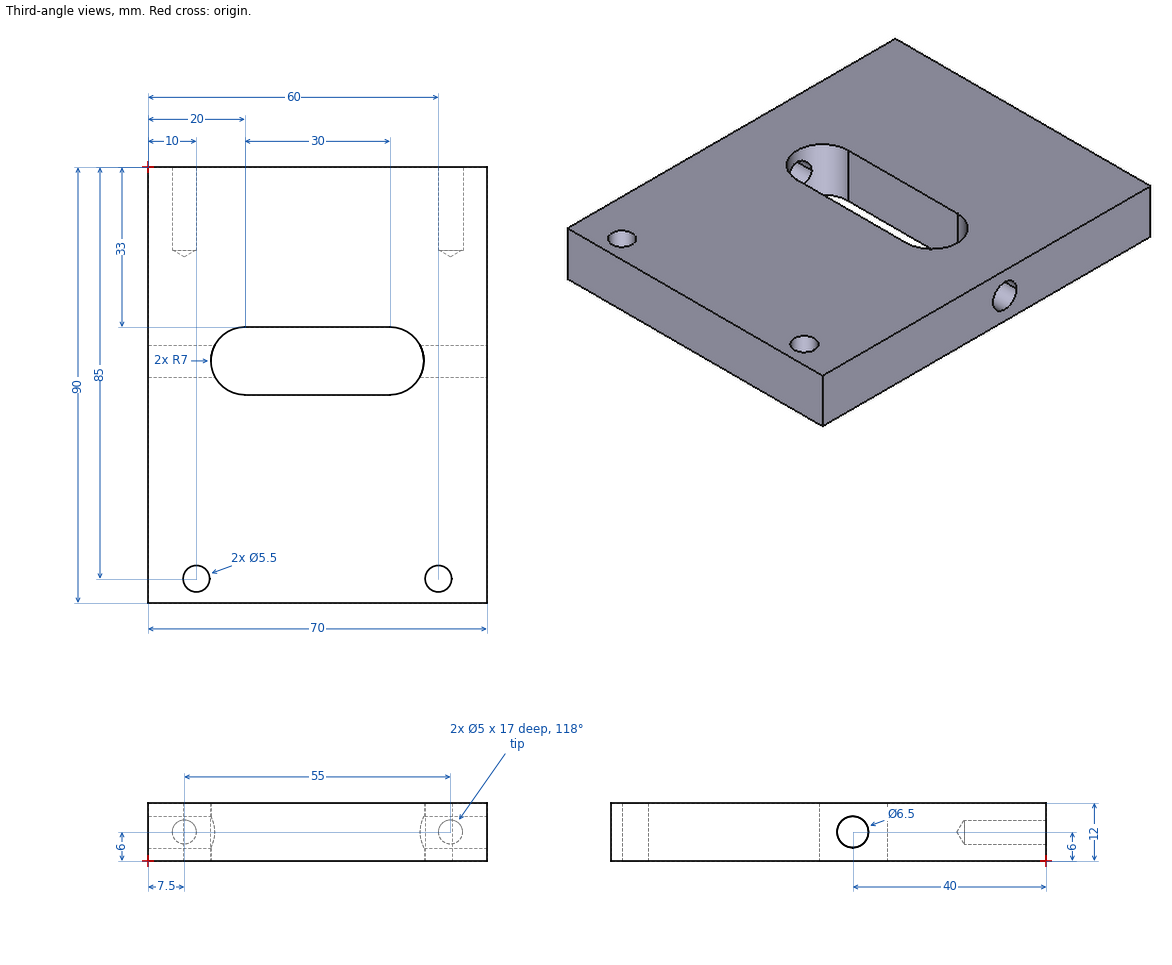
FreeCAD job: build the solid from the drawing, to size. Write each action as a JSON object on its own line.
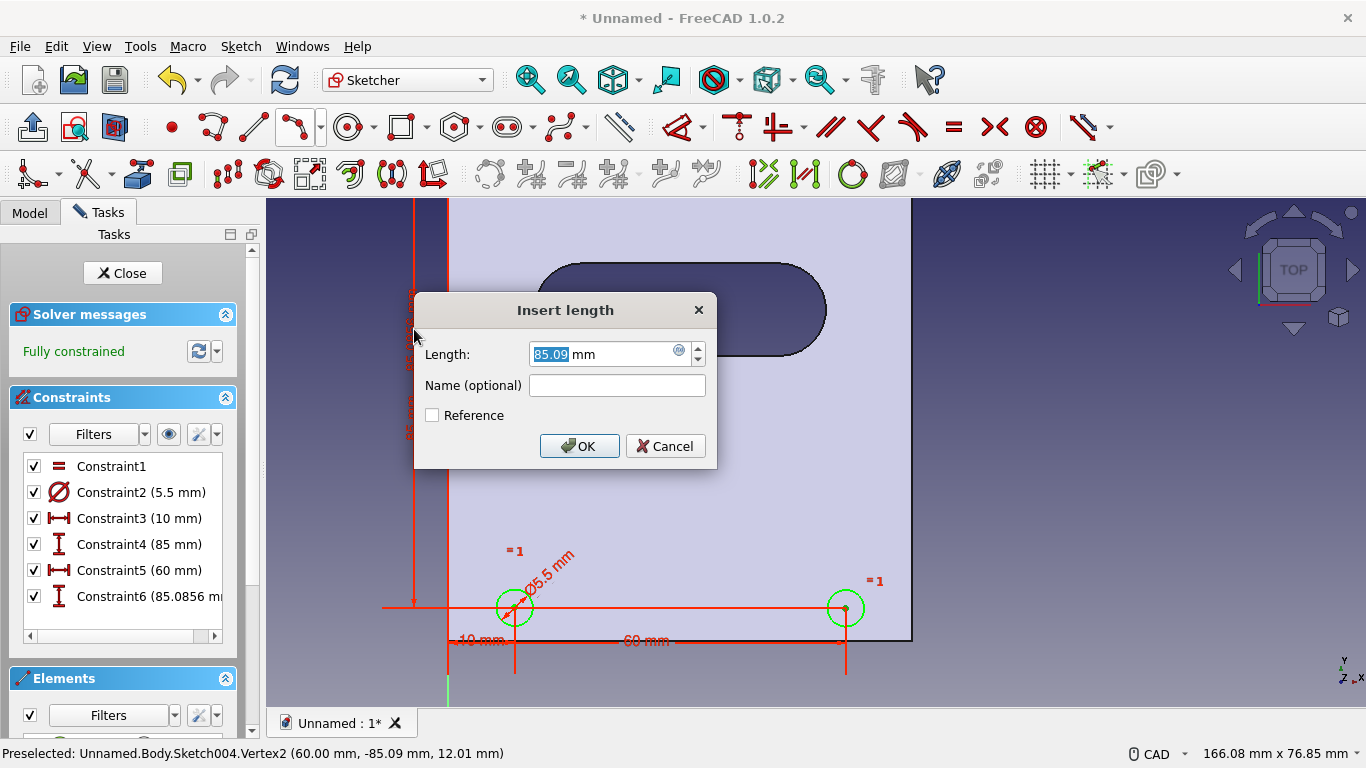
{"action": "type", "text": "85"}
{"action": "key", "text": "Return"}
{"action": "key", "text": "Escape"}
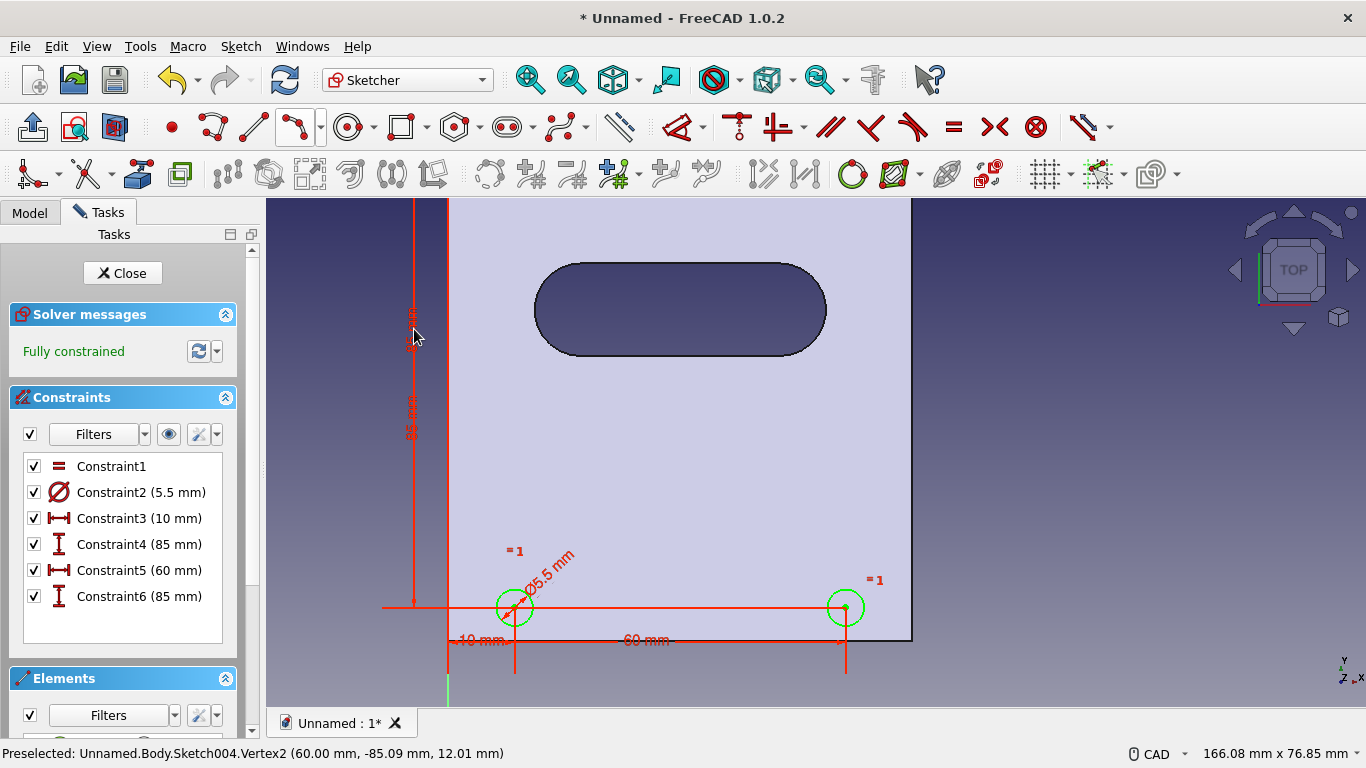
{"action": "left_click", "coordinate": [123, 273]}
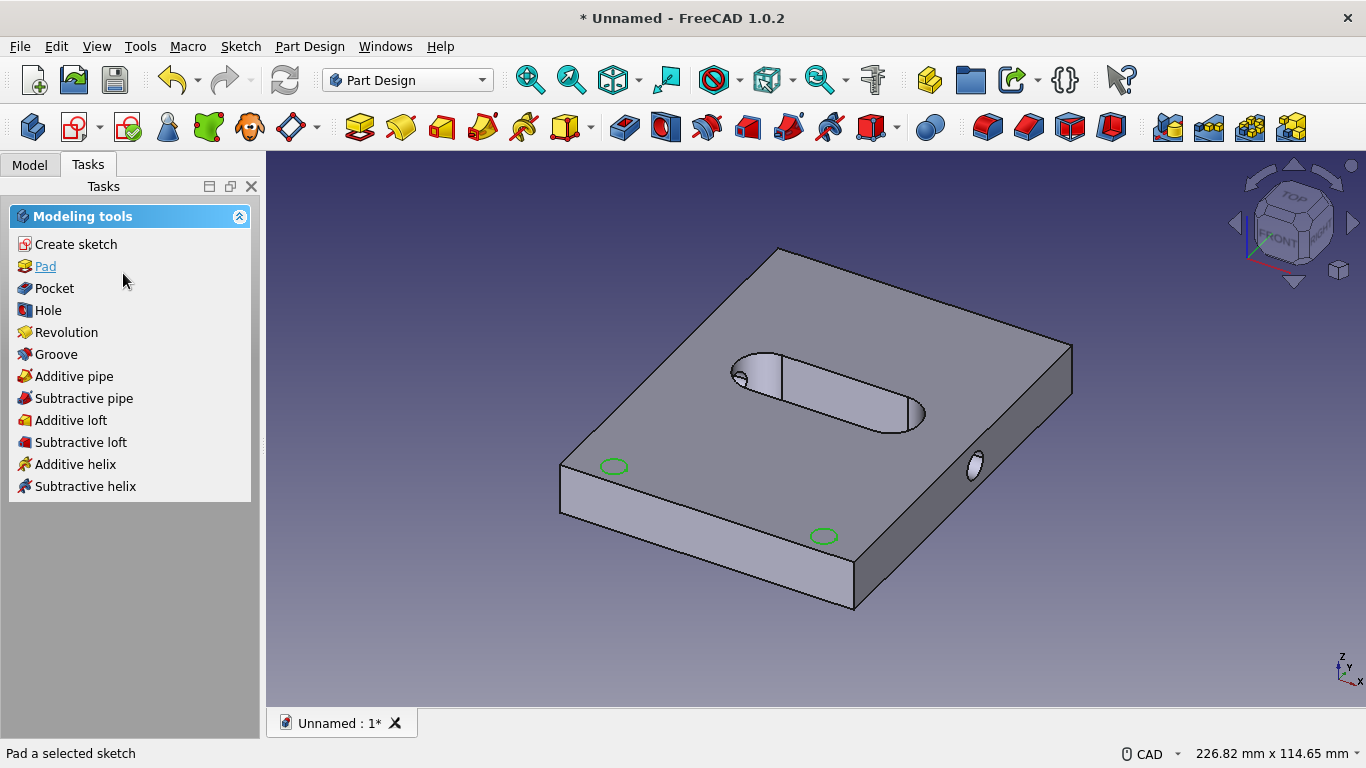
{"action": "left_click", "coordinate": [625, 128]}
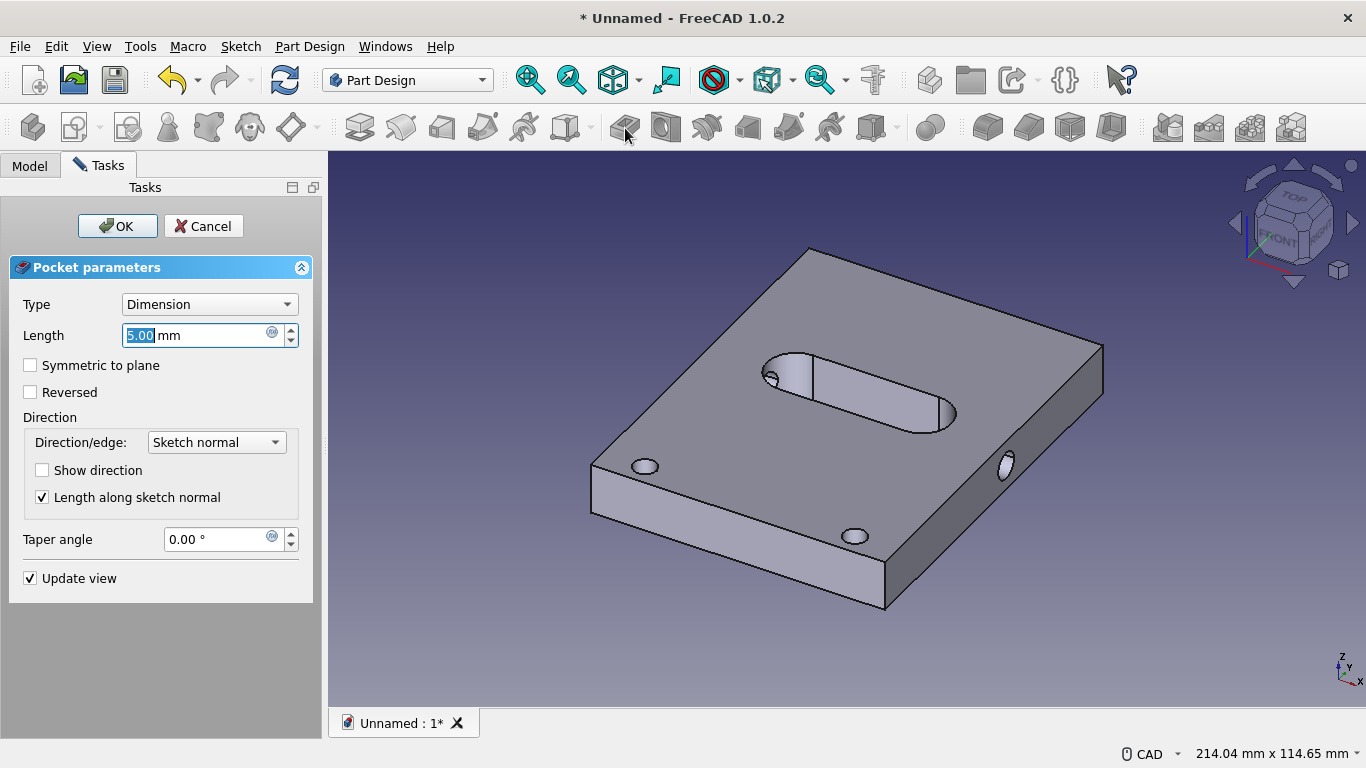
{"action": "left_click", "coordinate": [210, 304]}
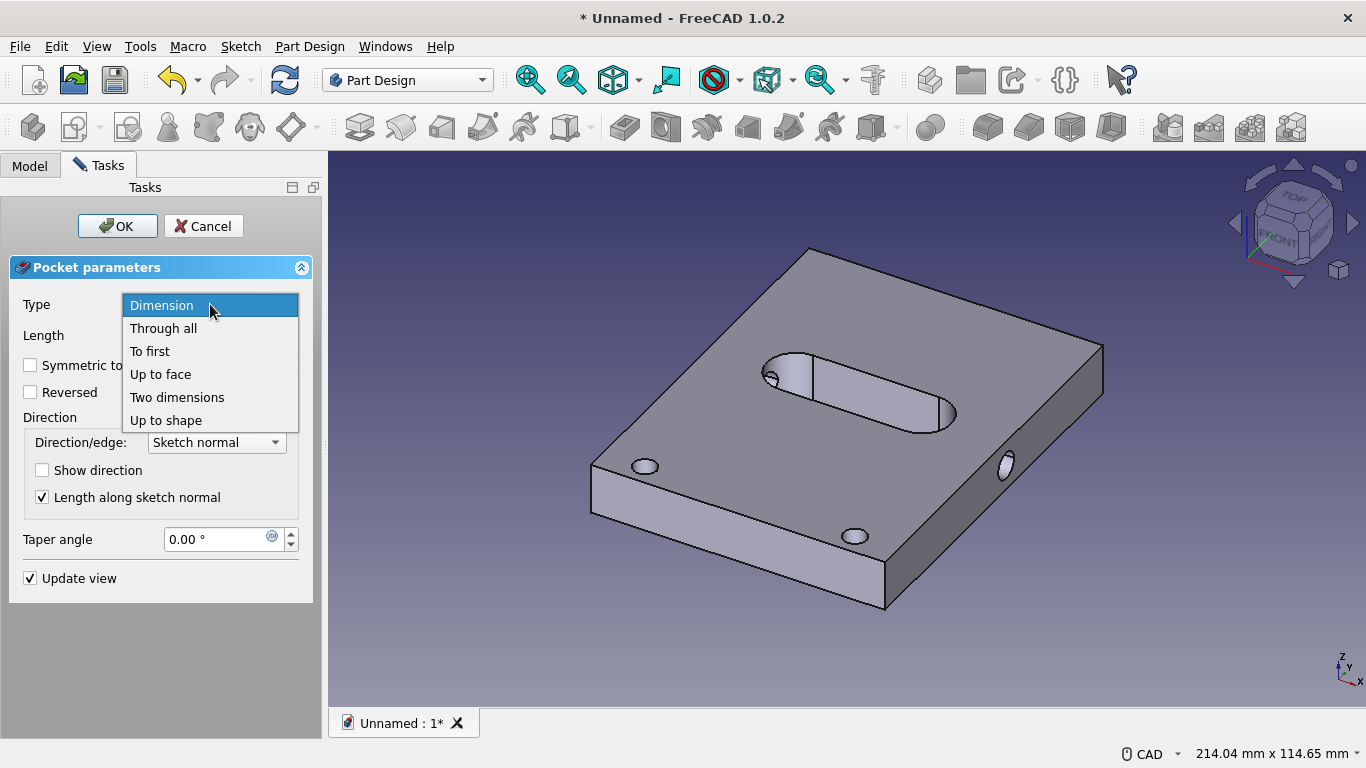
{"action": "left_click", "coordinate": [208, 328]}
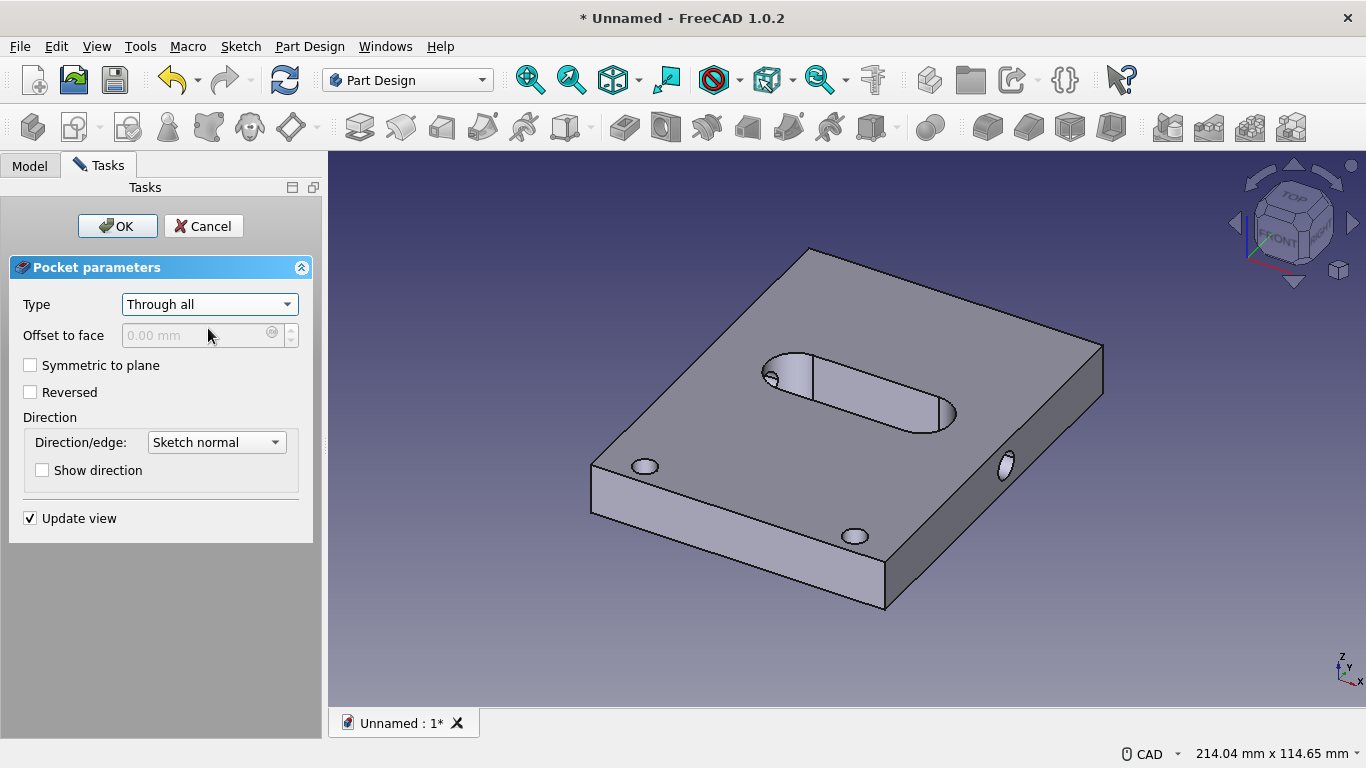
{"action": "left_click", "coordinate": [118, 226]}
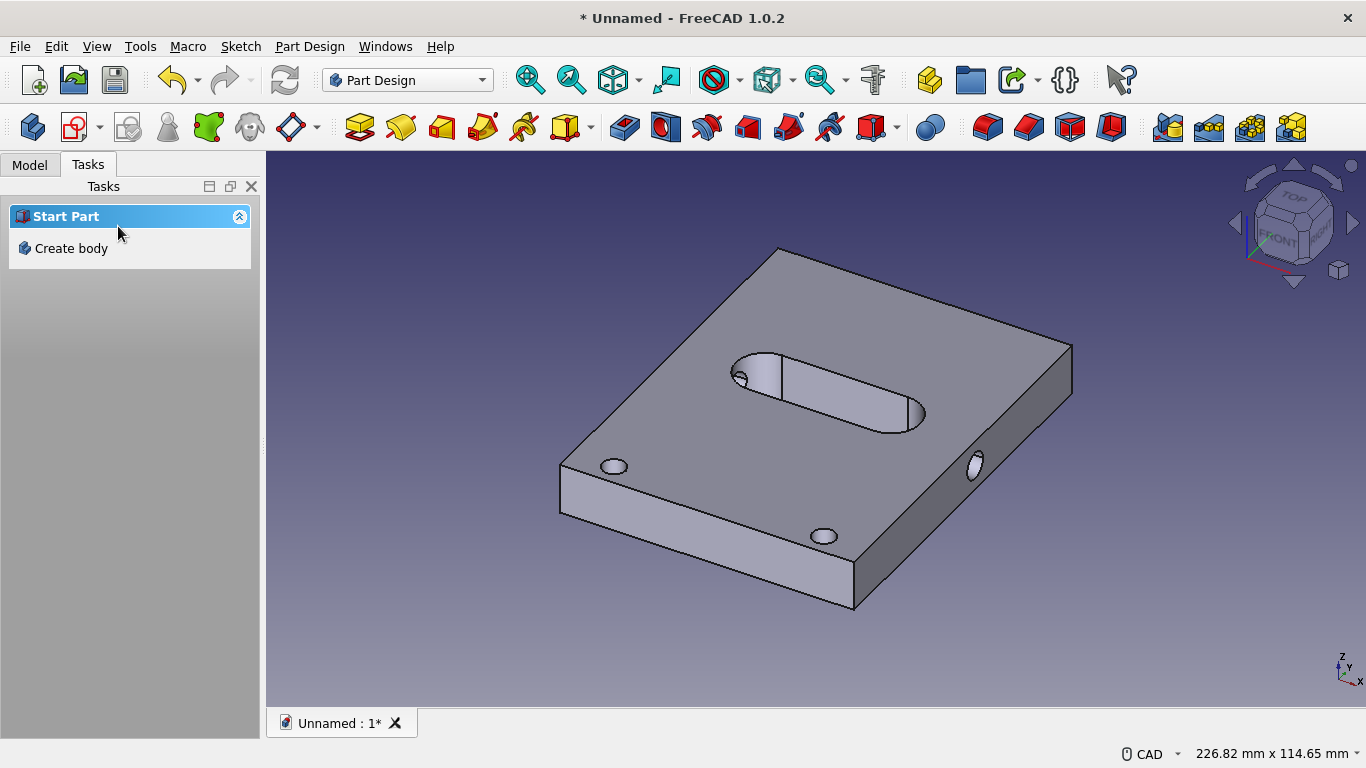
{"action": "key", "text": "0"}